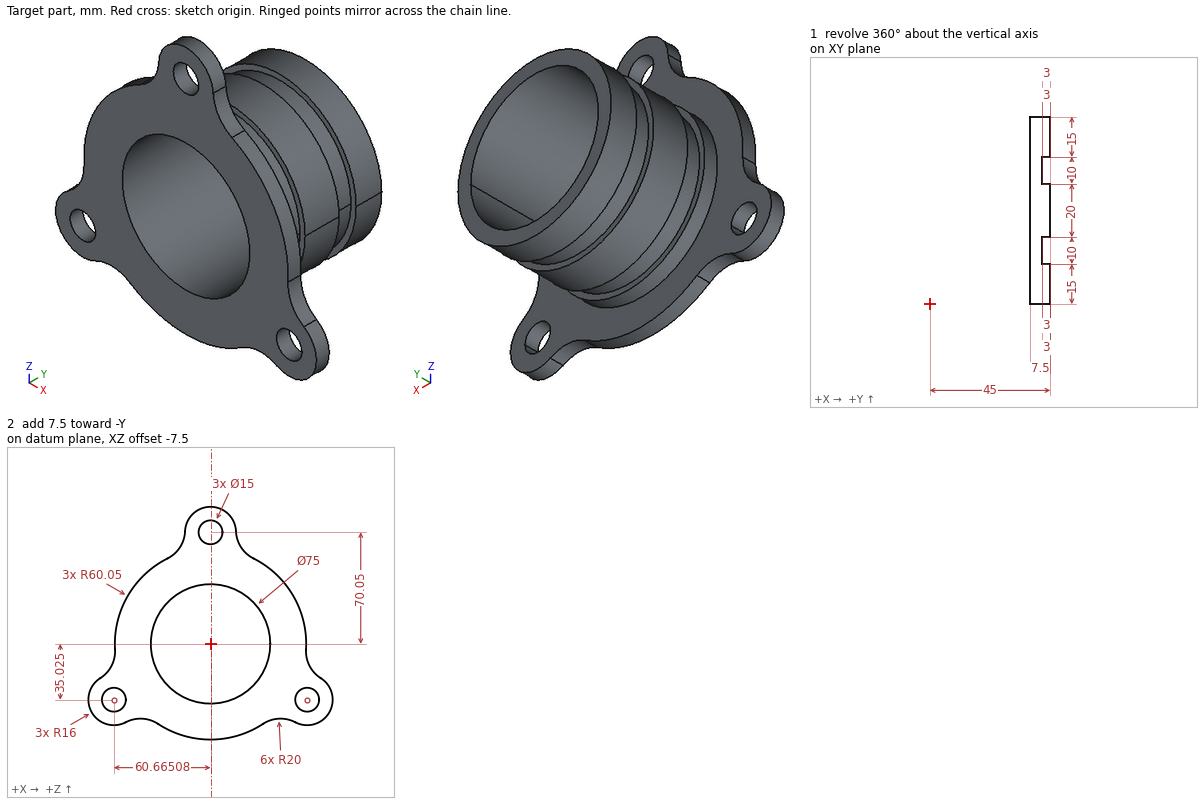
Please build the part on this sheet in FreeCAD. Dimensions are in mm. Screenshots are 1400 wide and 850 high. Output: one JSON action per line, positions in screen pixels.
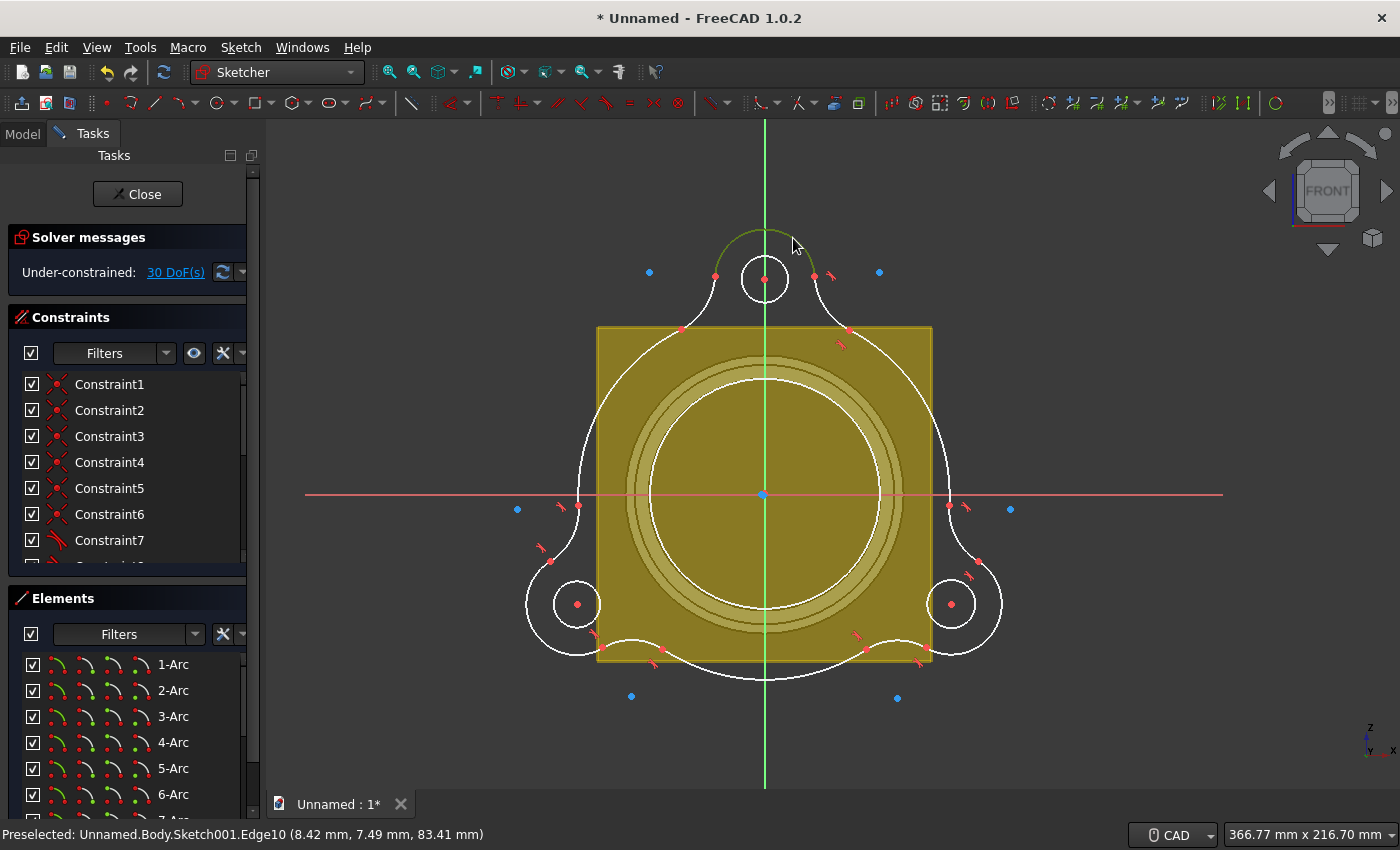
{"action": "left_click", "coordinate": [697, 318]}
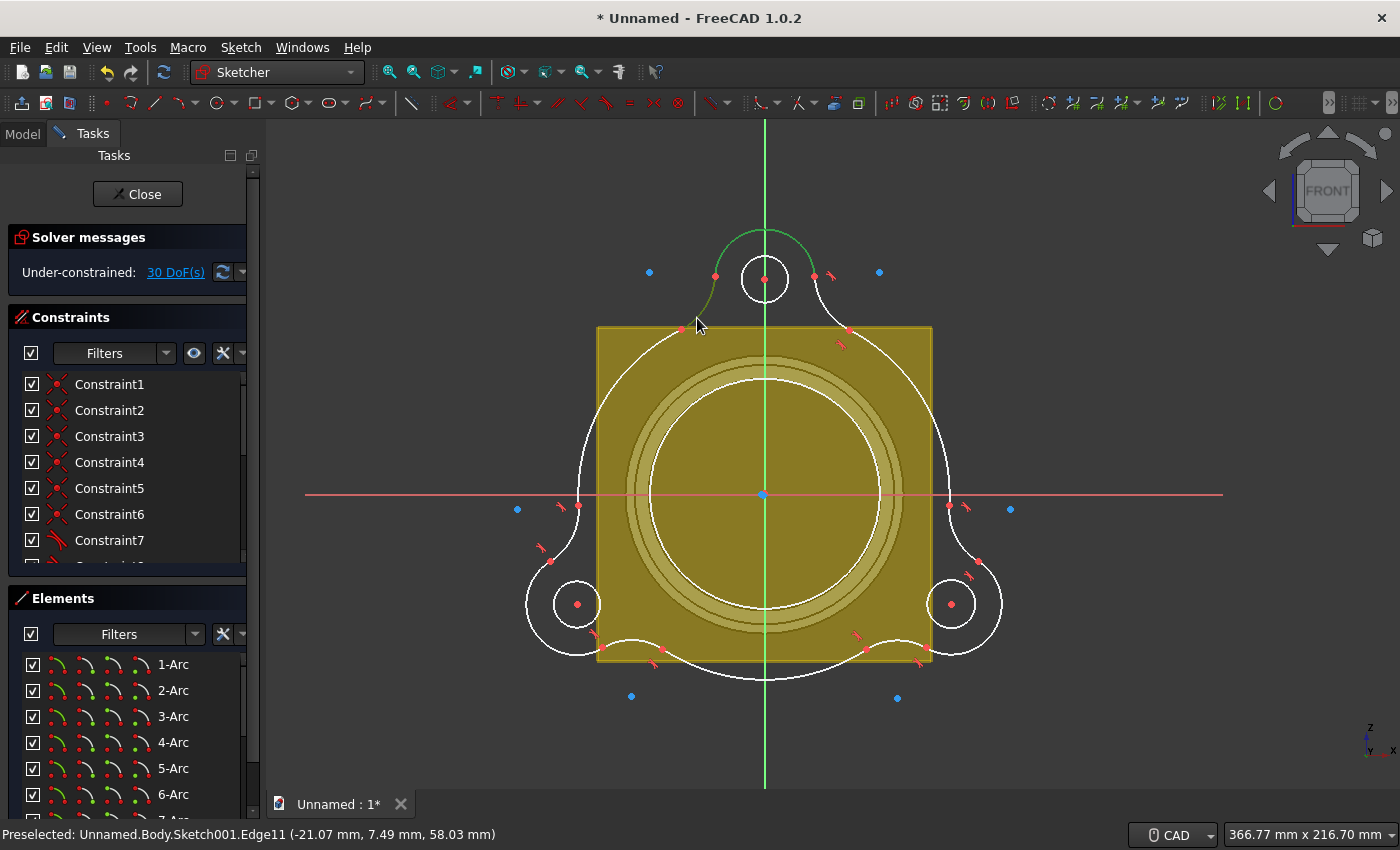
{"action": "left_click", "coordinate": [606, 104]}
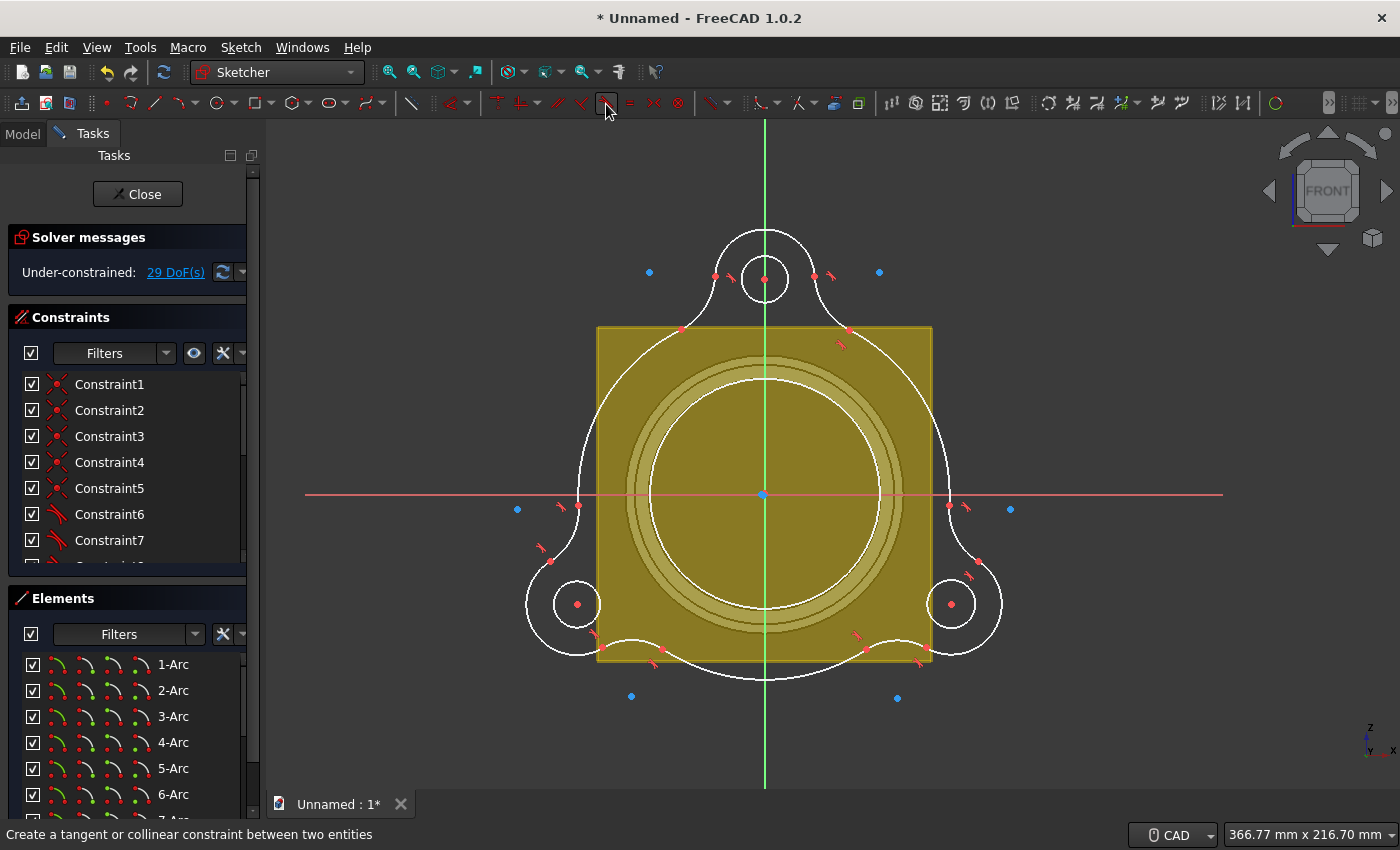
{"action": "left_click", "coordinate": [697, 318]}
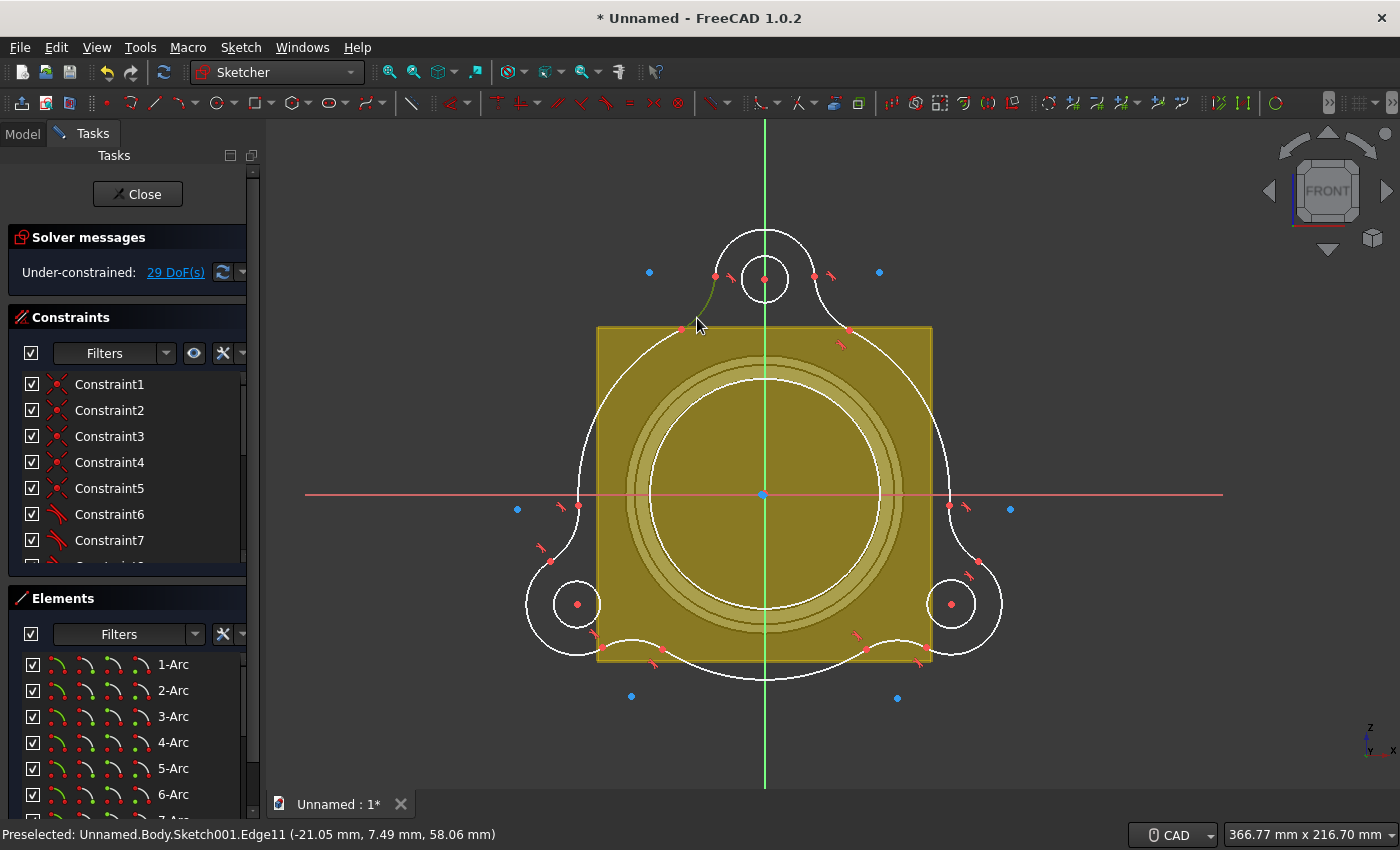
{"action": "left_click", "coordinate": [629, 368]}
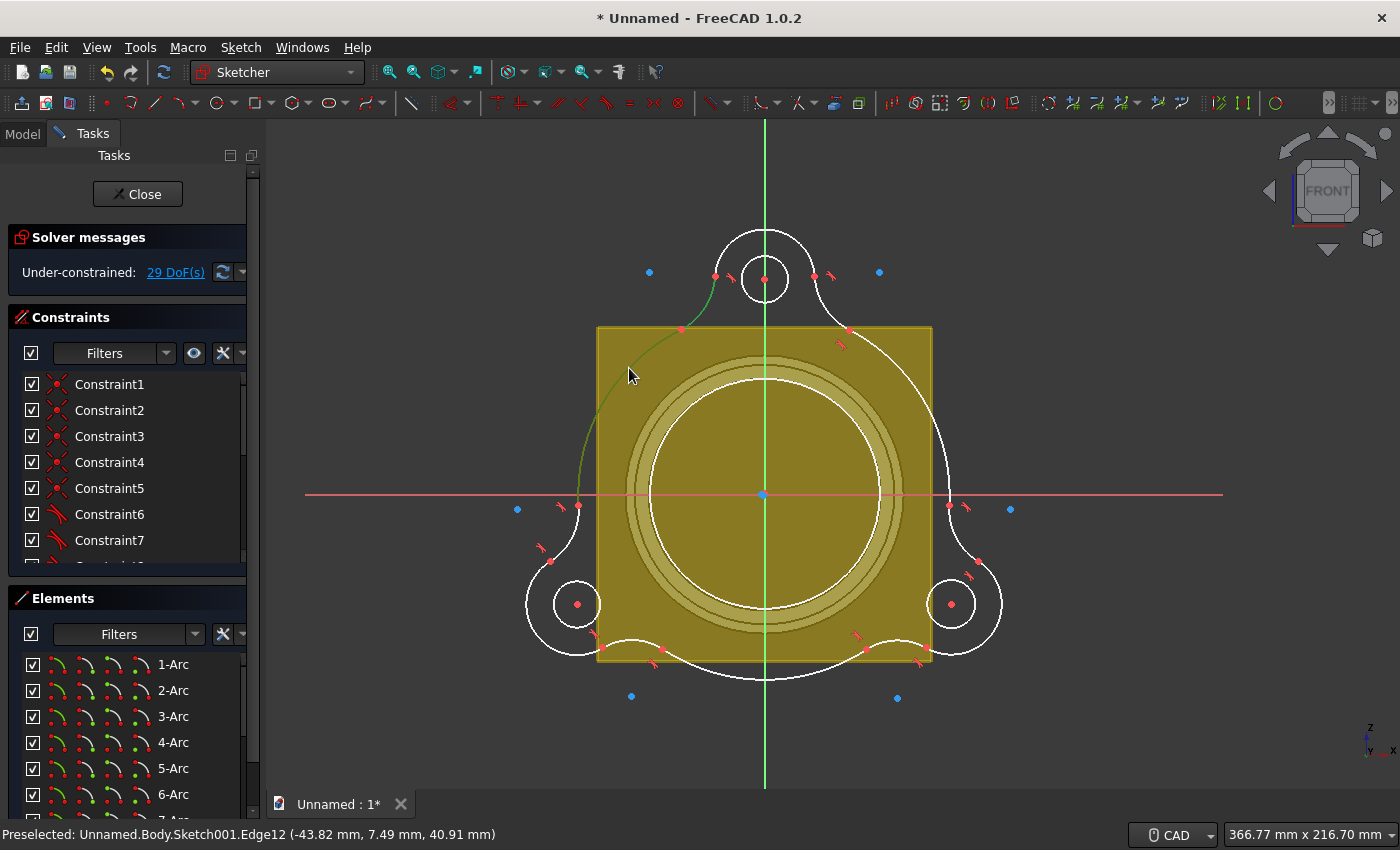
{"action": "left_click", "coordinate": [606, 104]}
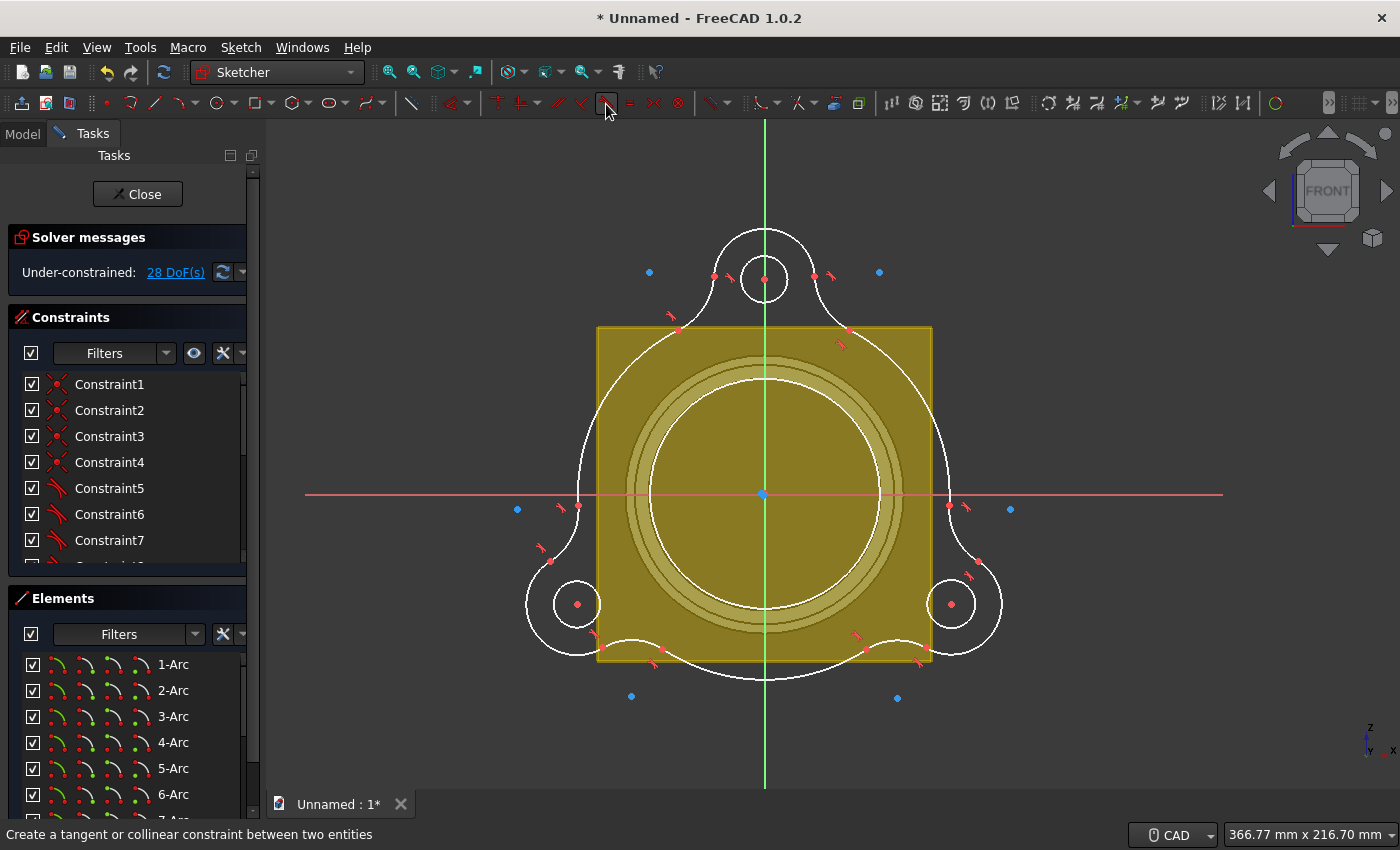
{"action": "left_click", "coordinate": [846, 412]}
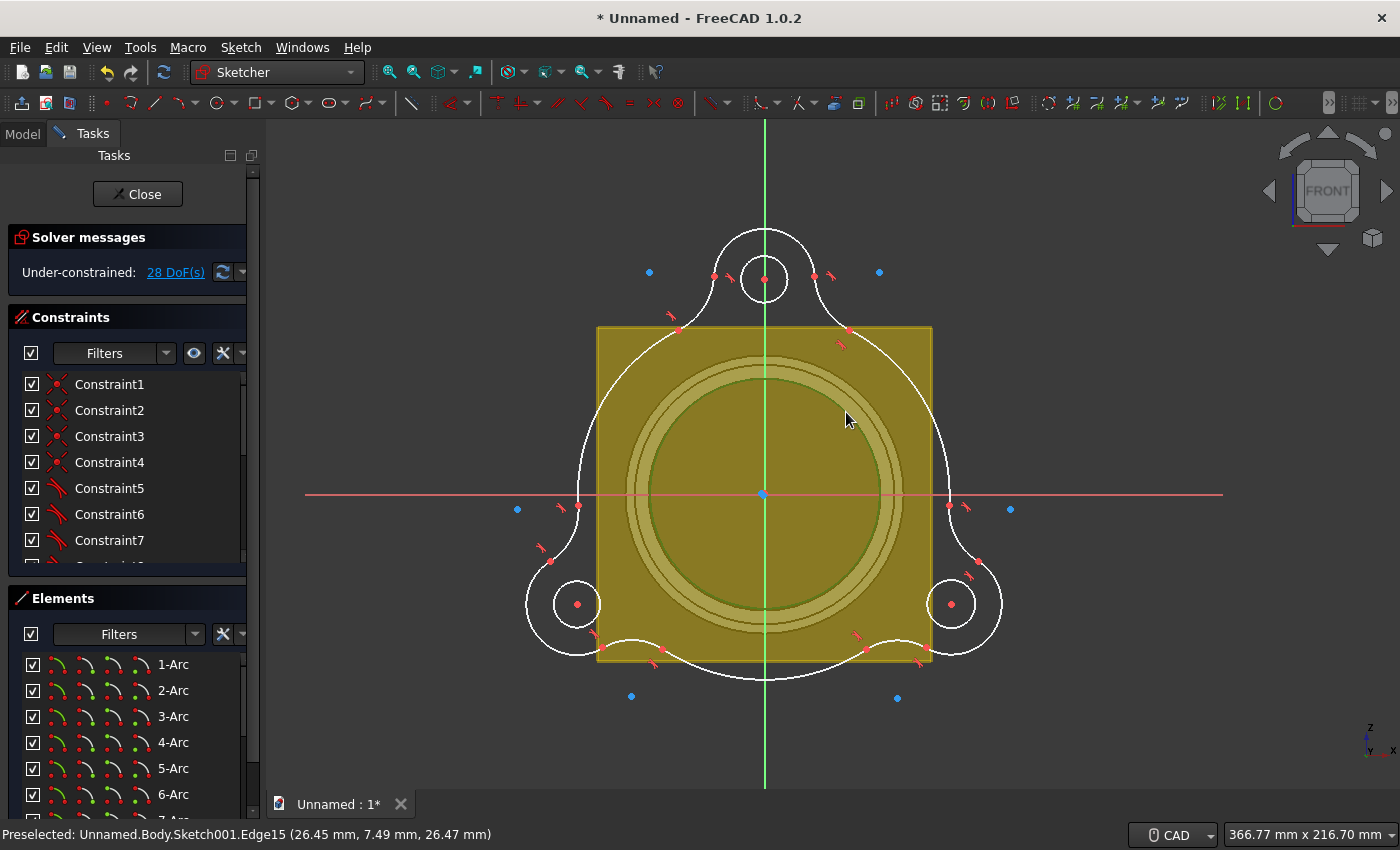
{"action": "left_click", "coordinate": [942, 442]}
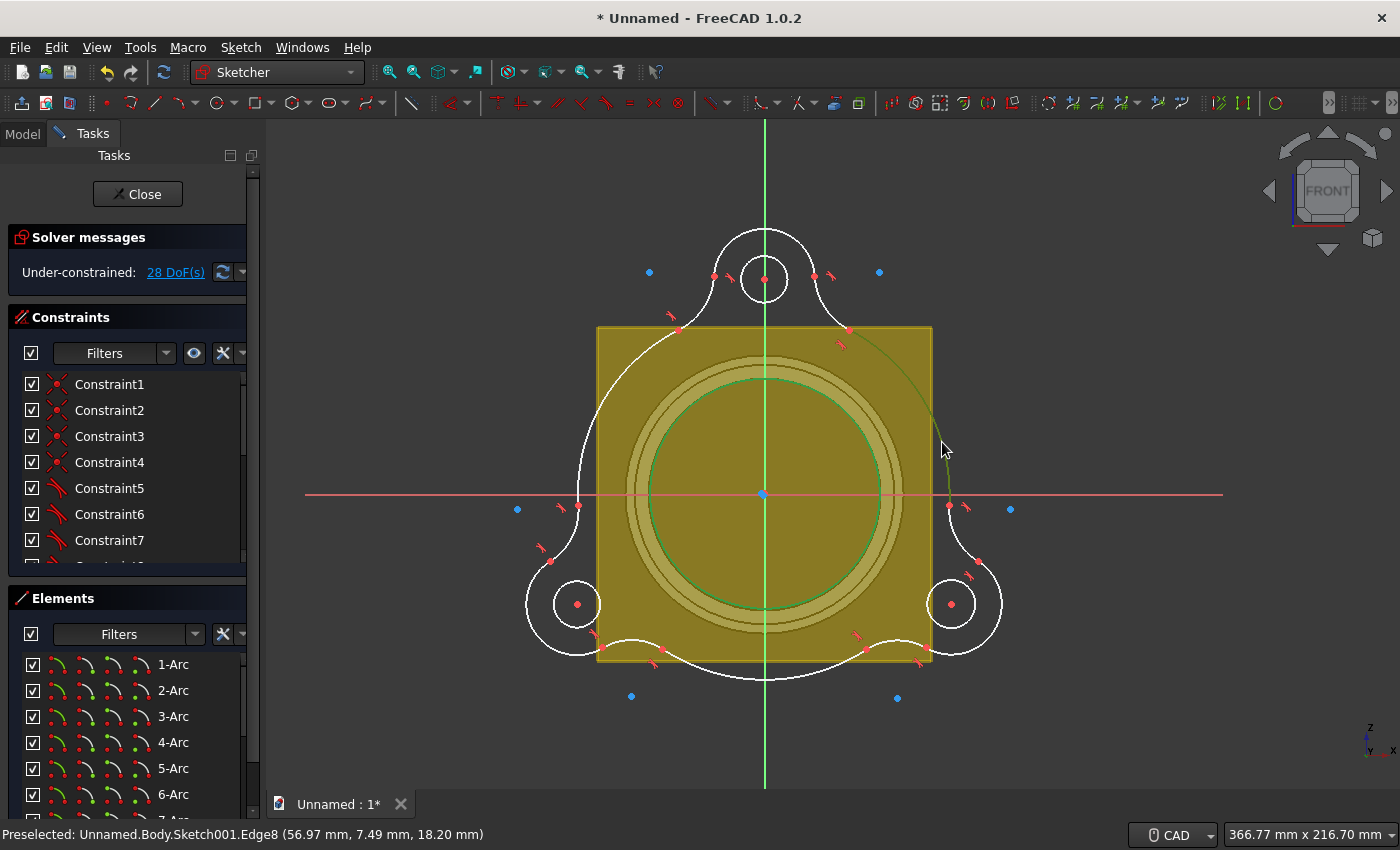
{"action": "left_click", "coordinate": [498, 104]}